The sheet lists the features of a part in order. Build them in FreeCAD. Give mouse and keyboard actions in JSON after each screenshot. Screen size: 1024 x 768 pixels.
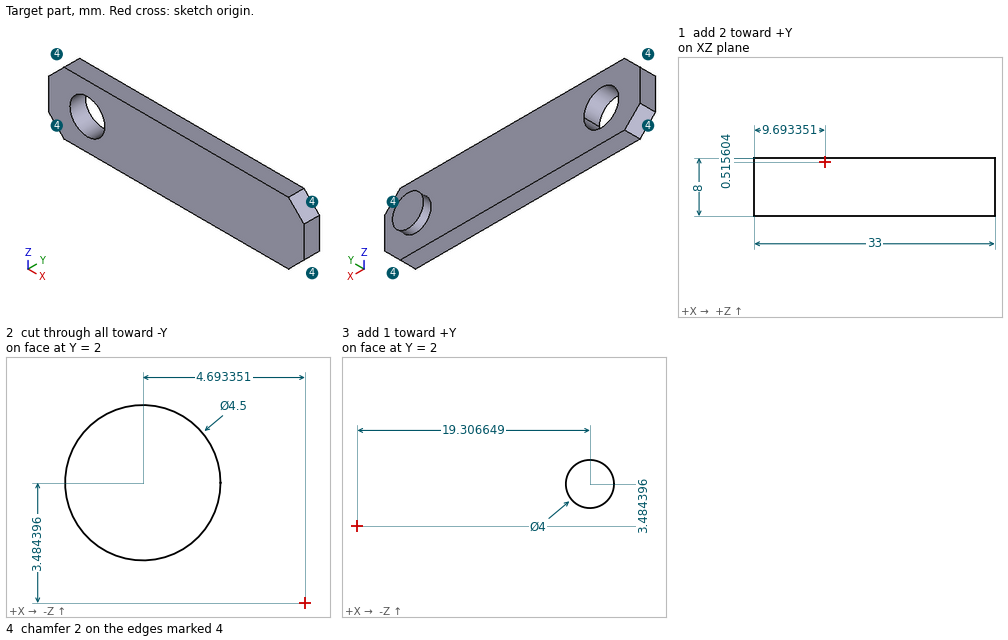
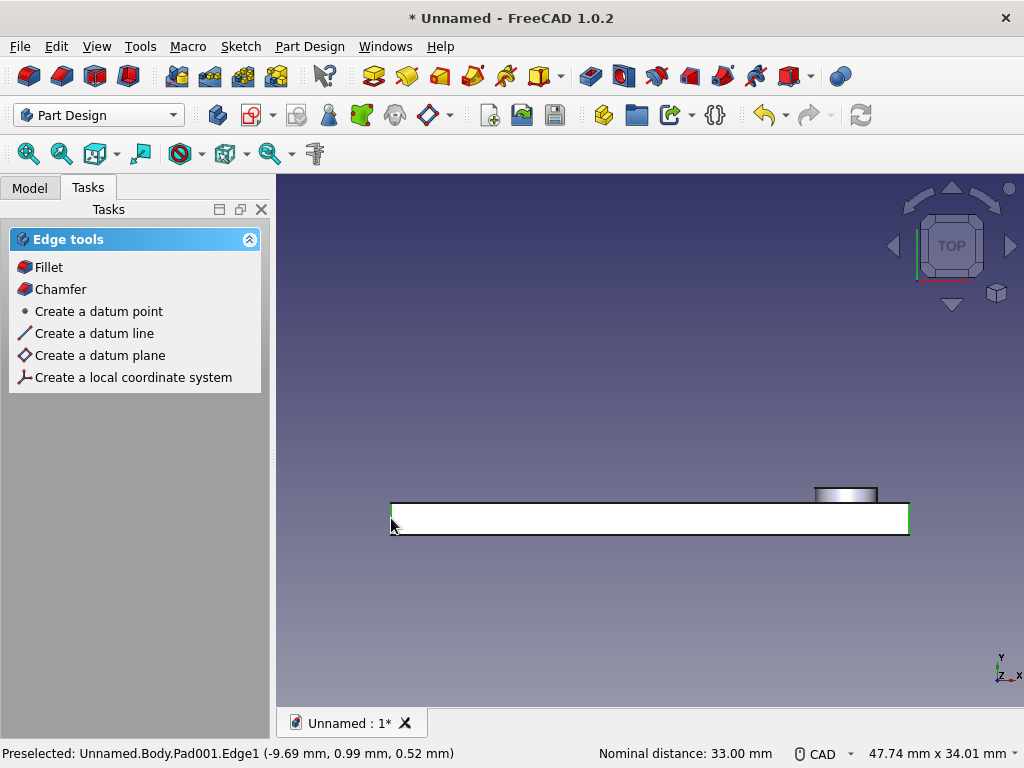
{"action": "key", "text": "1"}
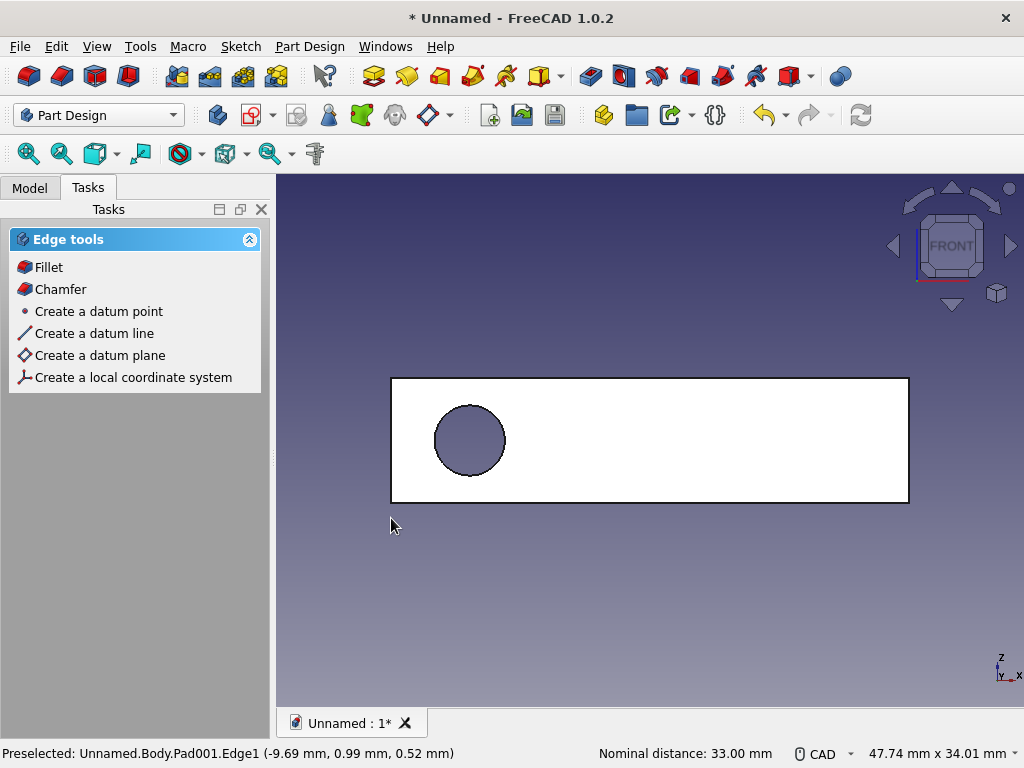
{"action": "key", "text": "3"}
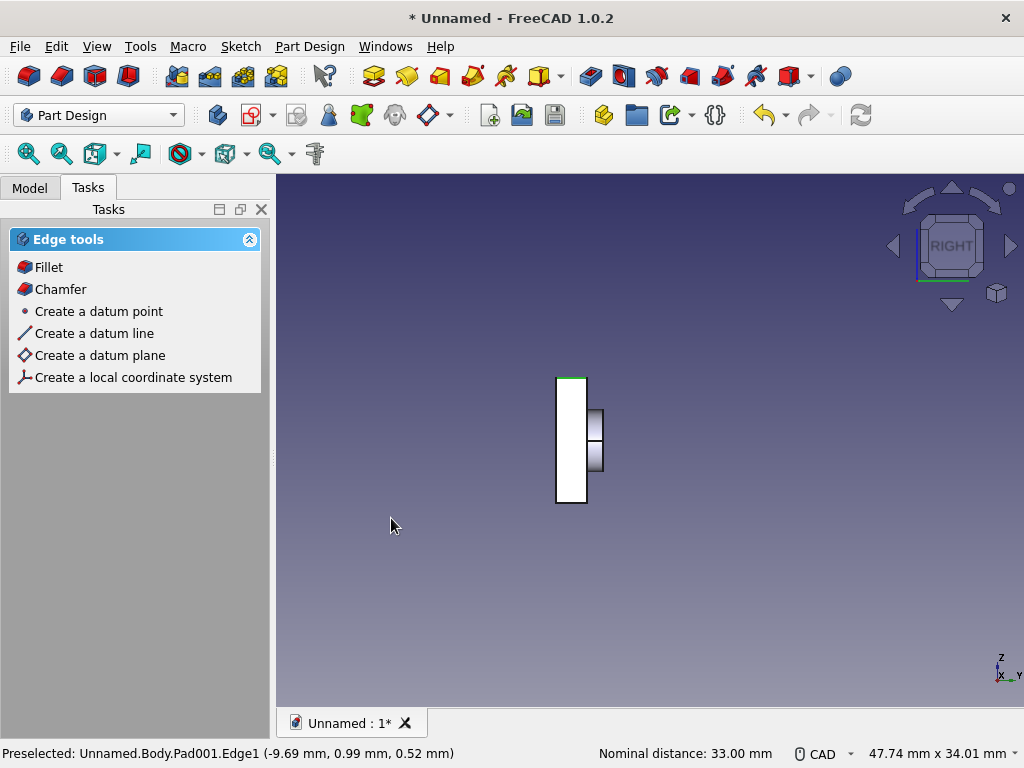
{"action": "left_click", "coordinate": [29, 154]}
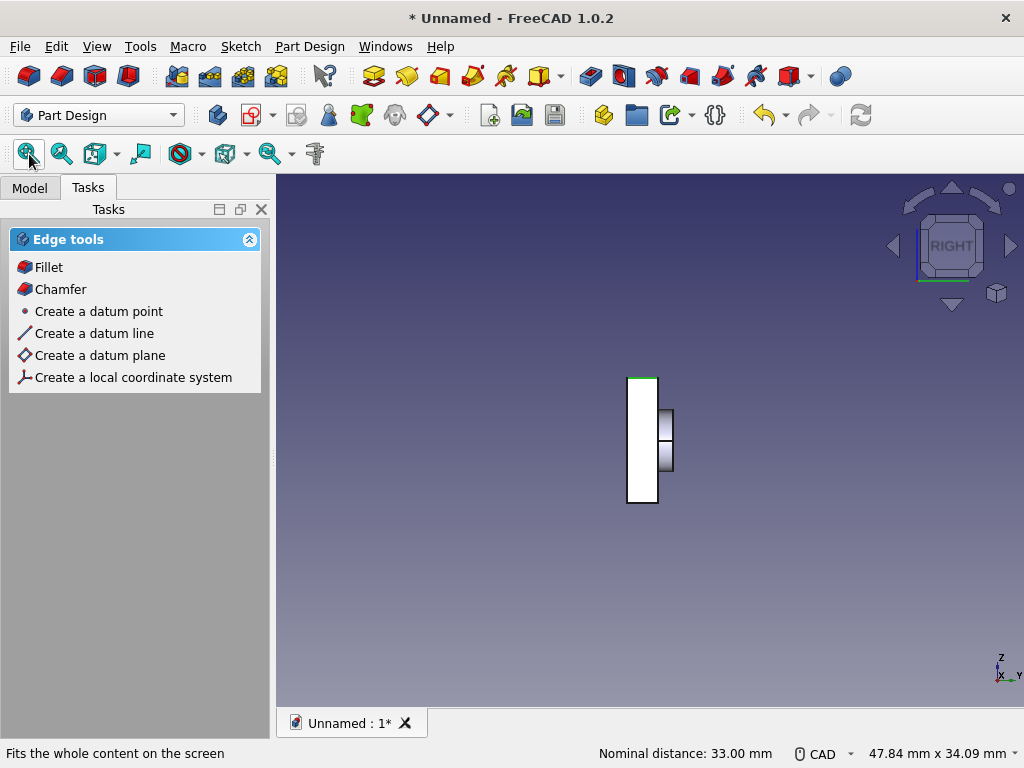
{"action": "left_click", "coordinate": [642, 502], "text": "ctrl"}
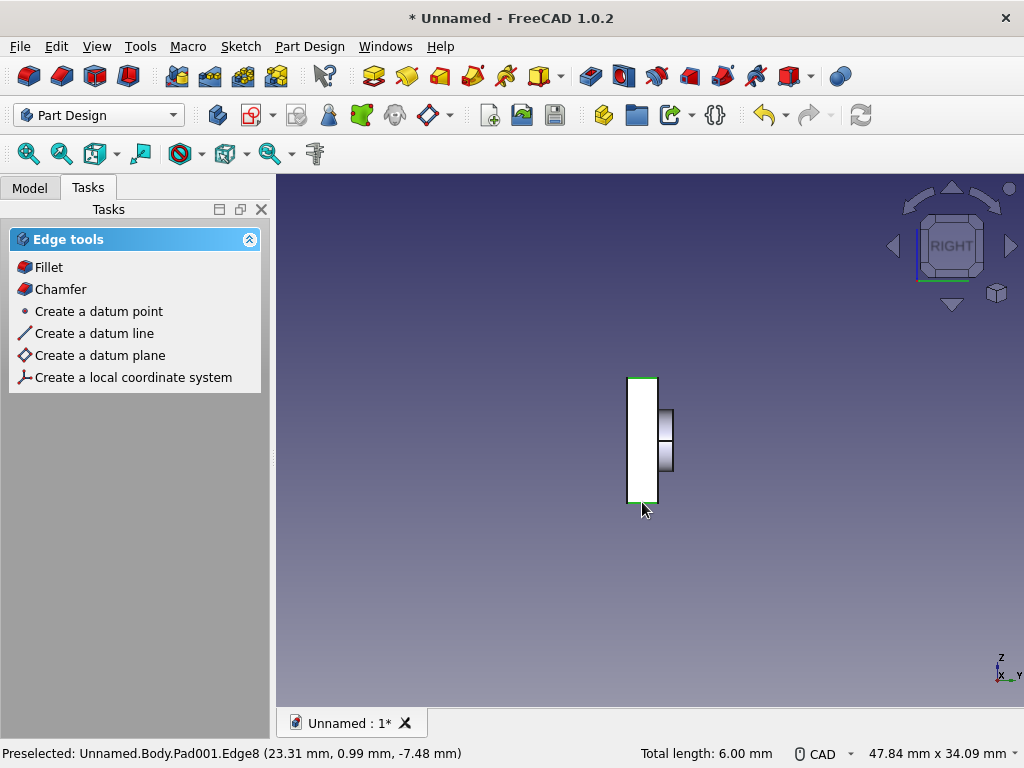
{"action": "key", "text": "5"}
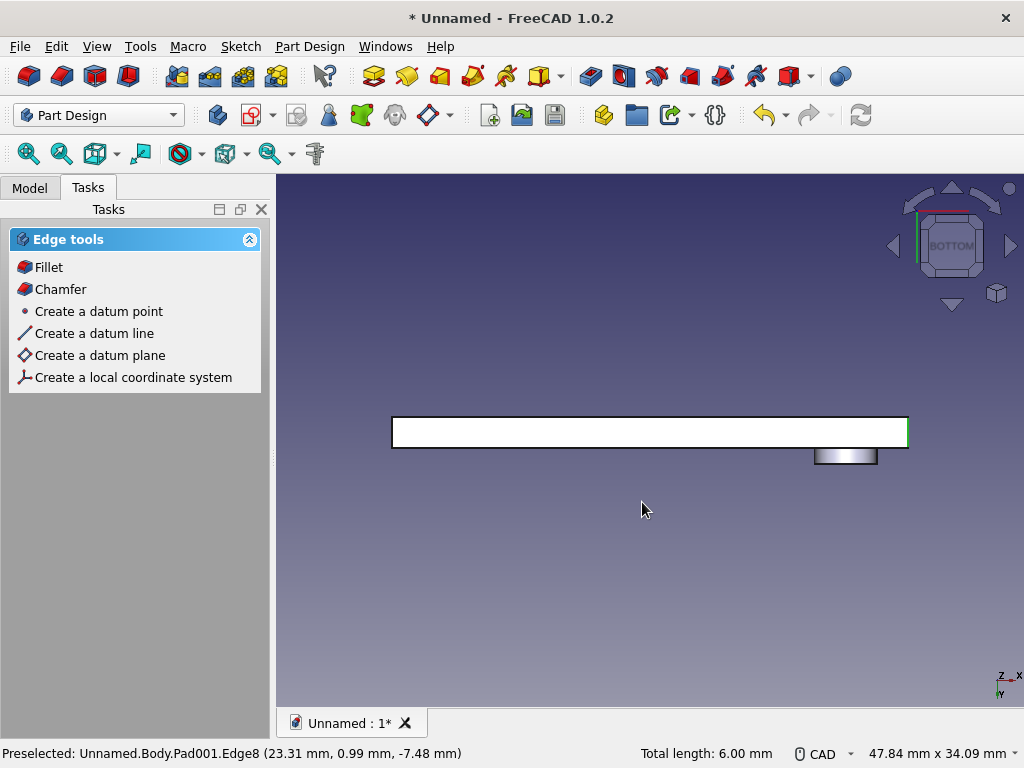
{"action": "left_click", "coordinate": [392, 432], "text": "ctrl"}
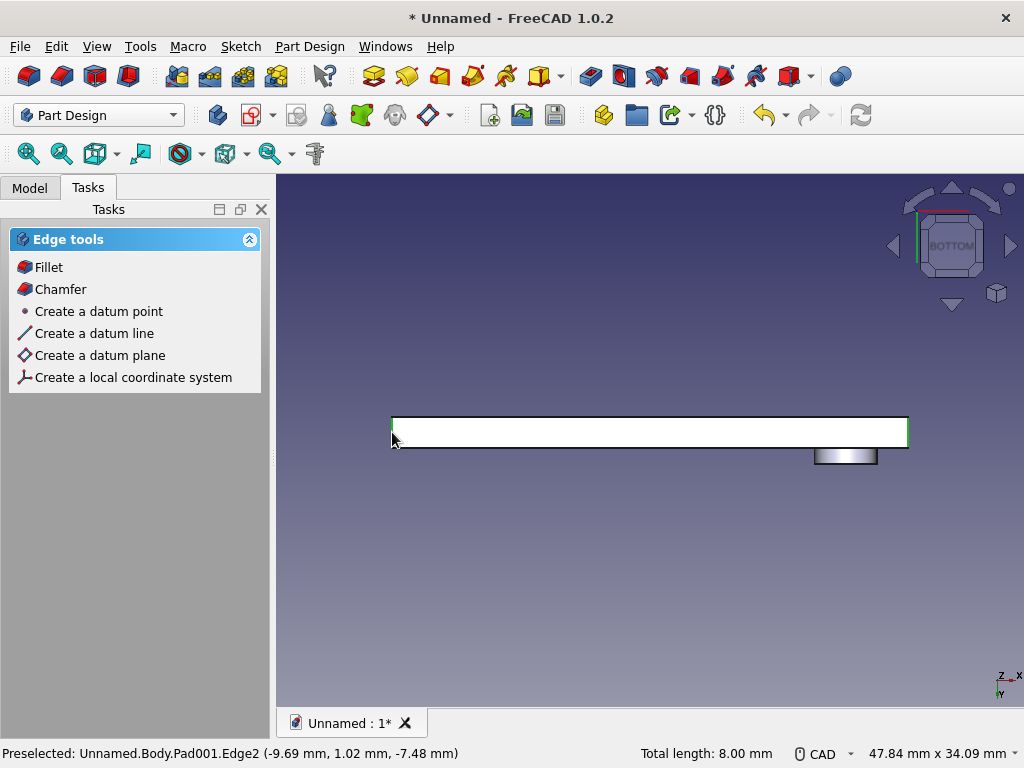
{"action": "left_click", "coordinate": [62, 76]}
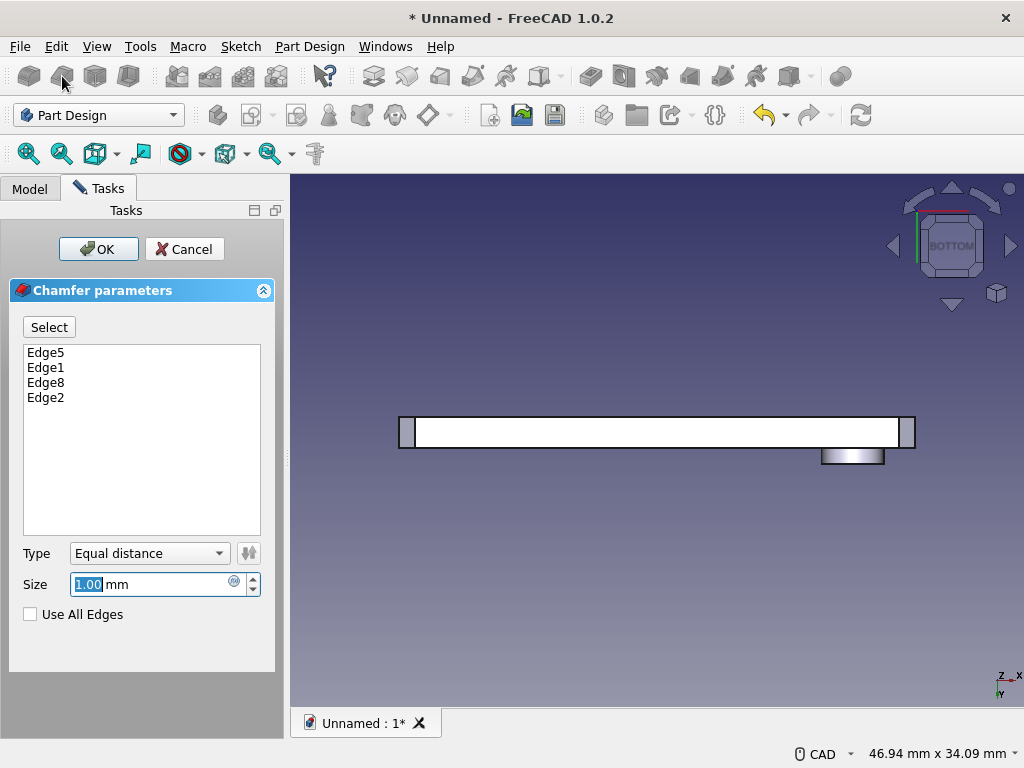
{"action": "type", "text": "2"}
{"action": "key", "text": "Tab"}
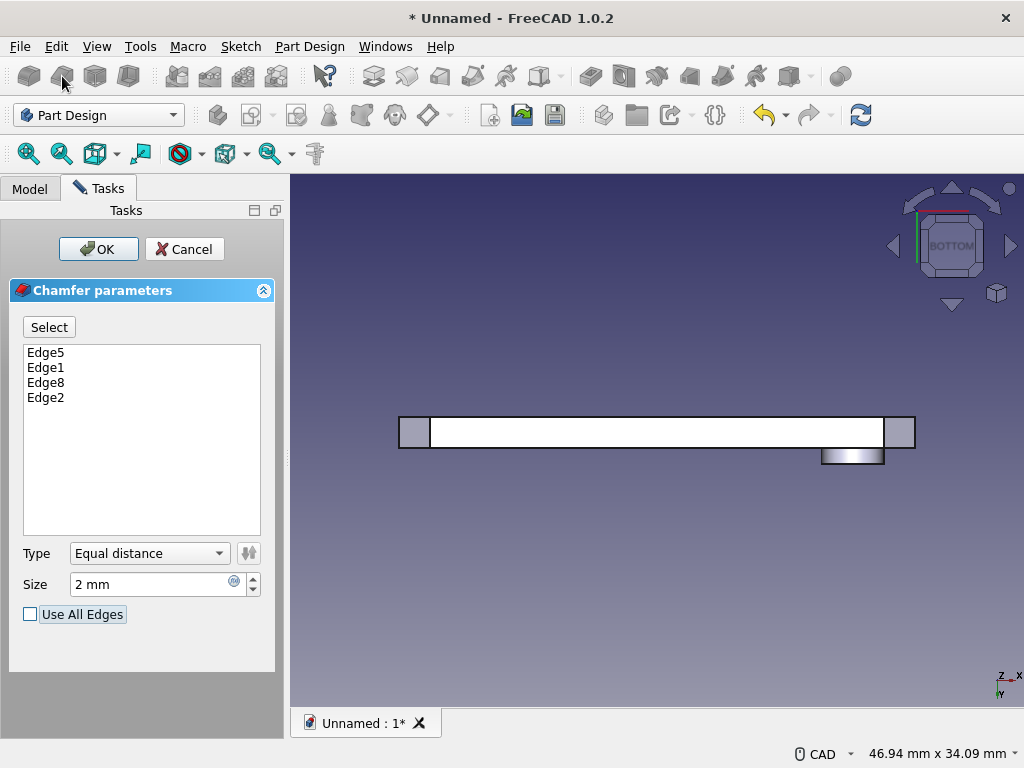
{"action": "left_click", "coordinate": [99, 249]}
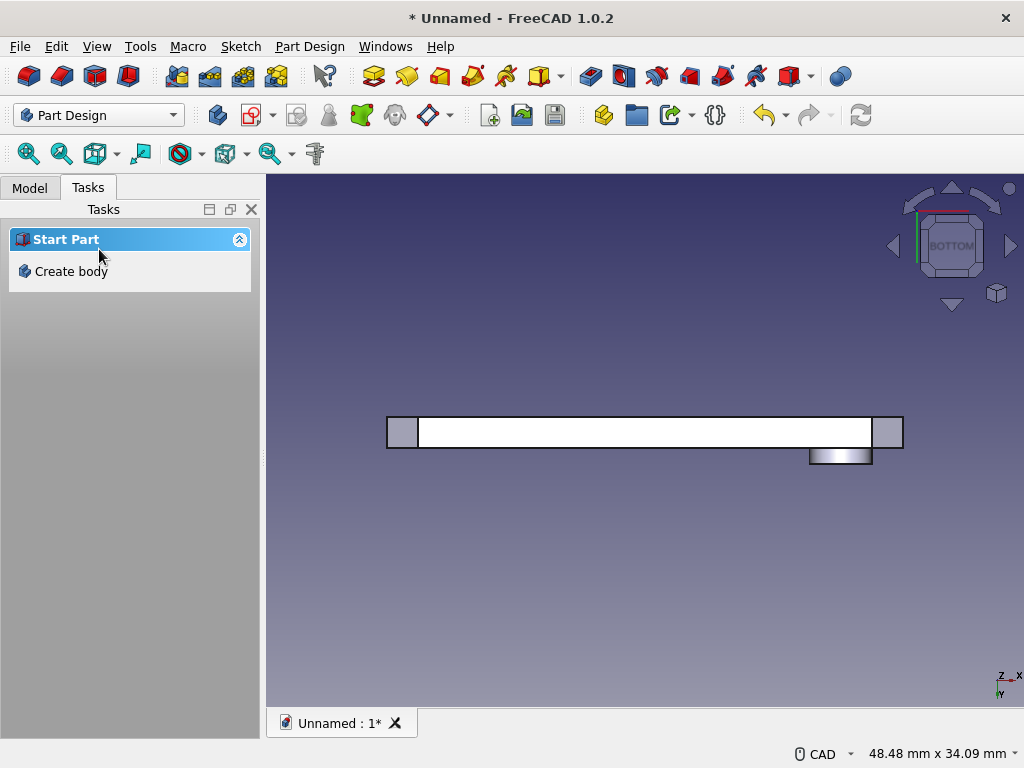
{"action": "key", "text": "0"}